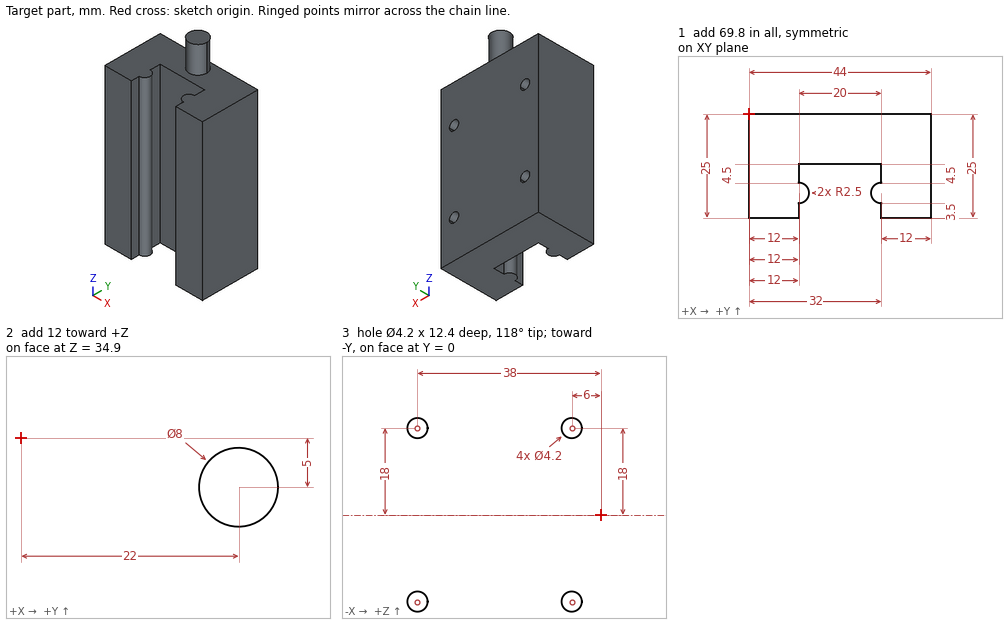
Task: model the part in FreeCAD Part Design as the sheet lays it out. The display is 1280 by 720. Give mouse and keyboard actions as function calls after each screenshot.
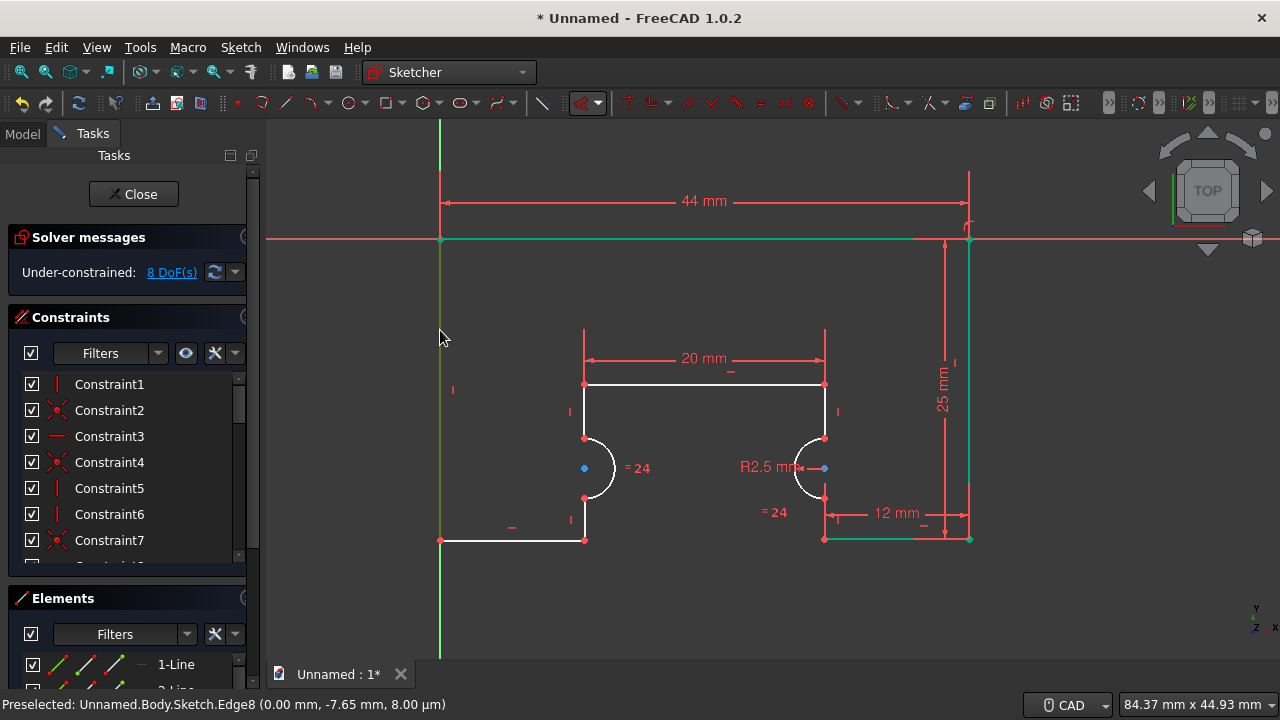
click(600, 104)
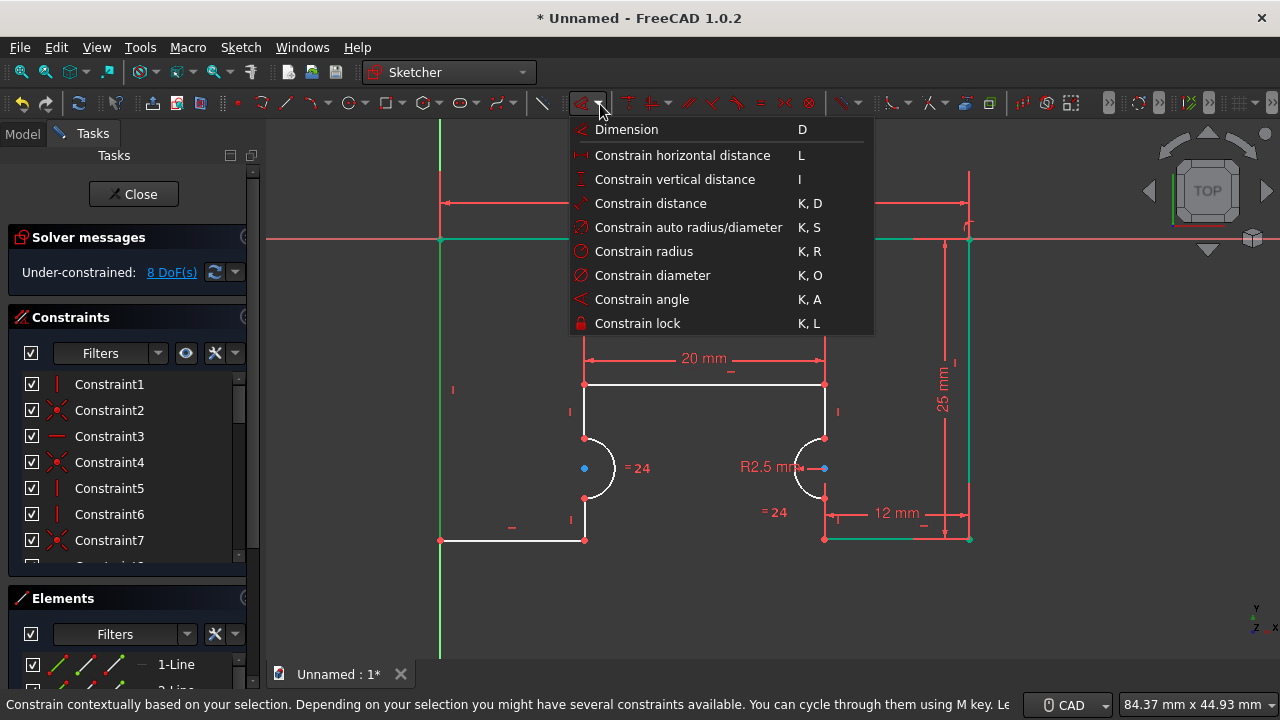
click(722, 179)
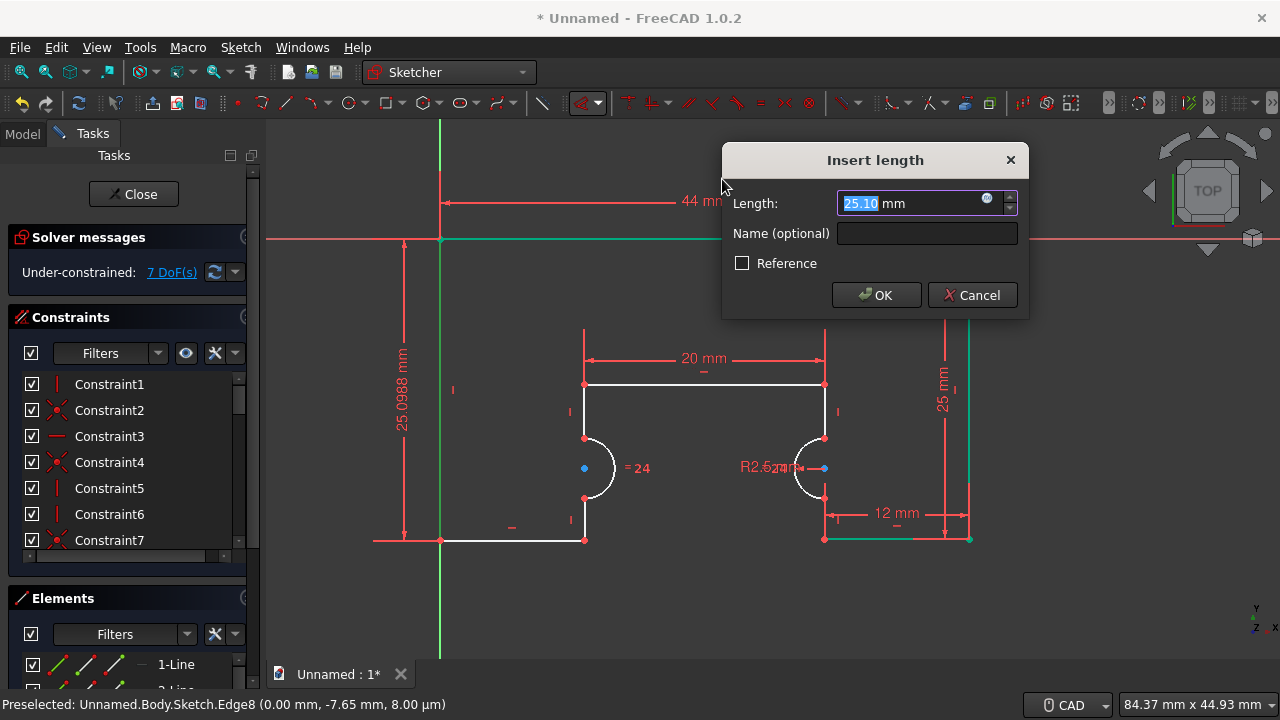
text(25)
key(Return)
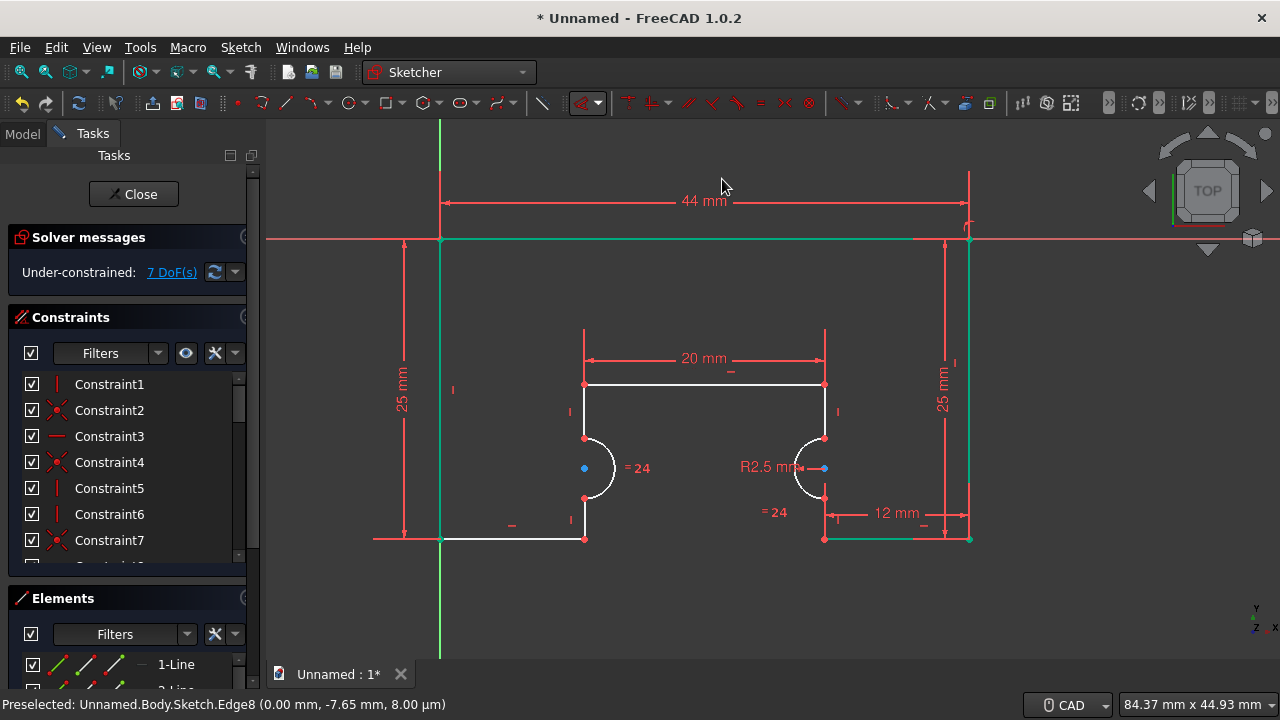
click(484, 539)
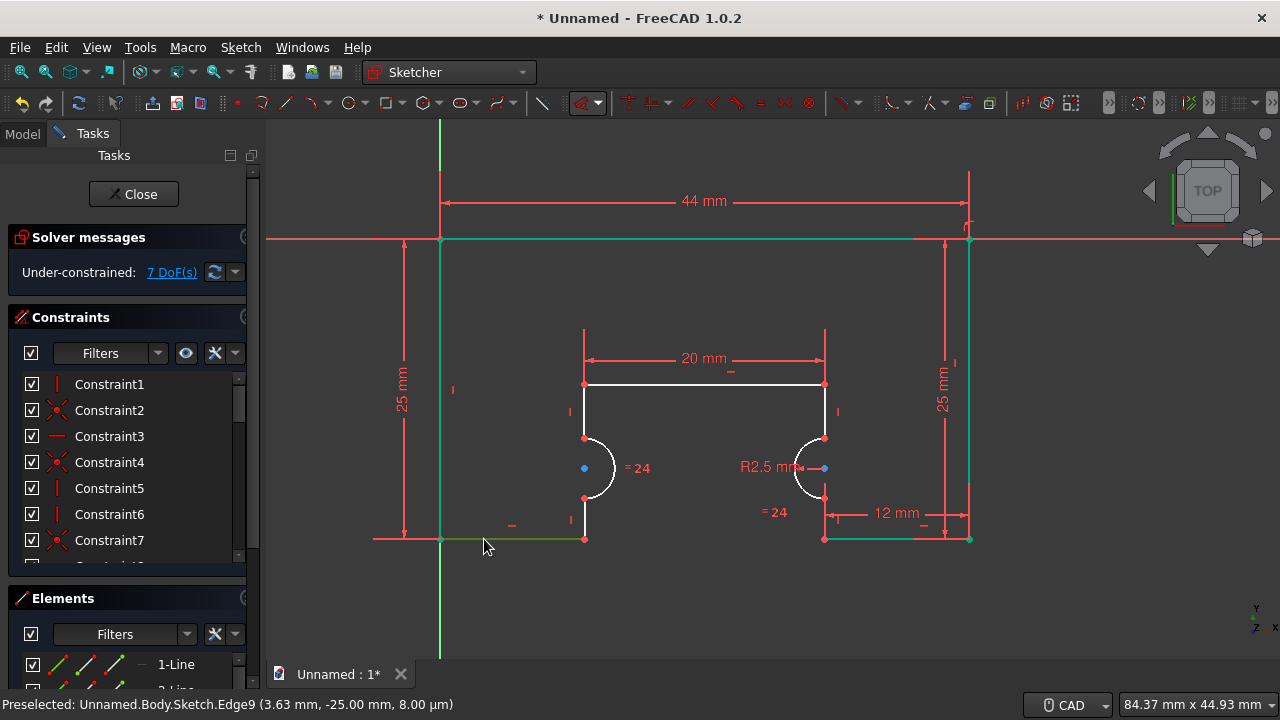
click(600, 104)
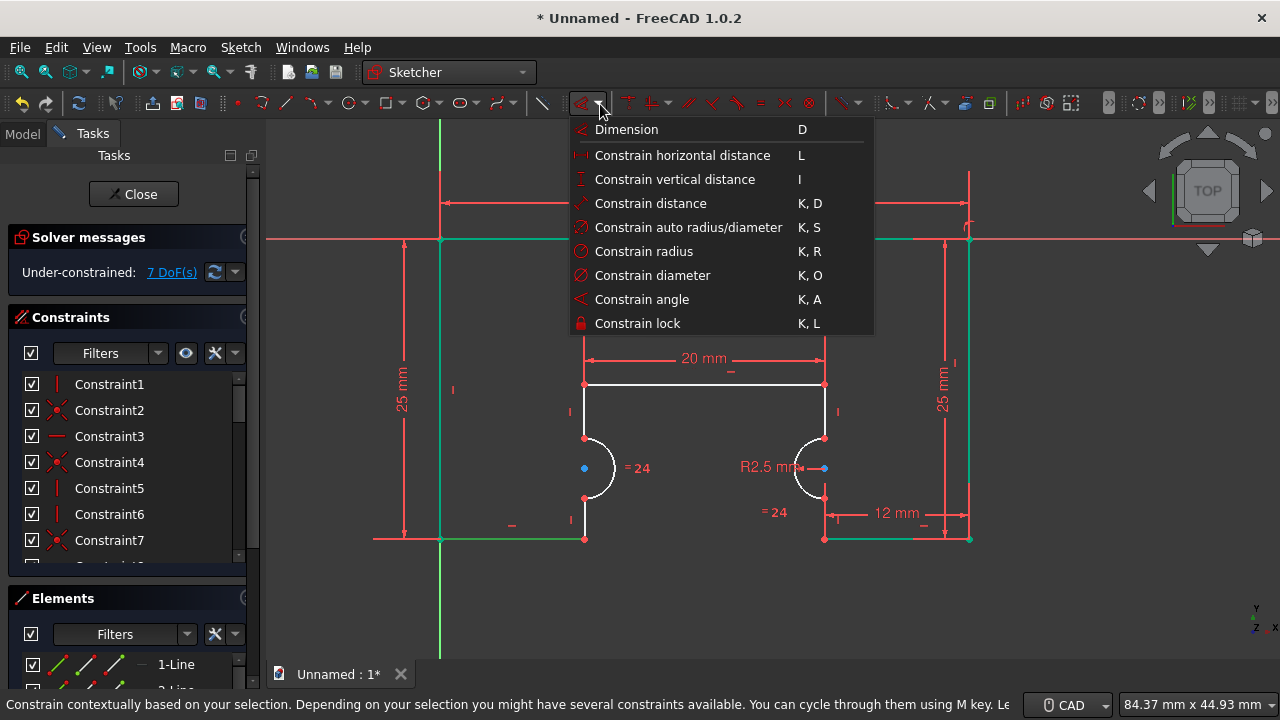
click(722, 155)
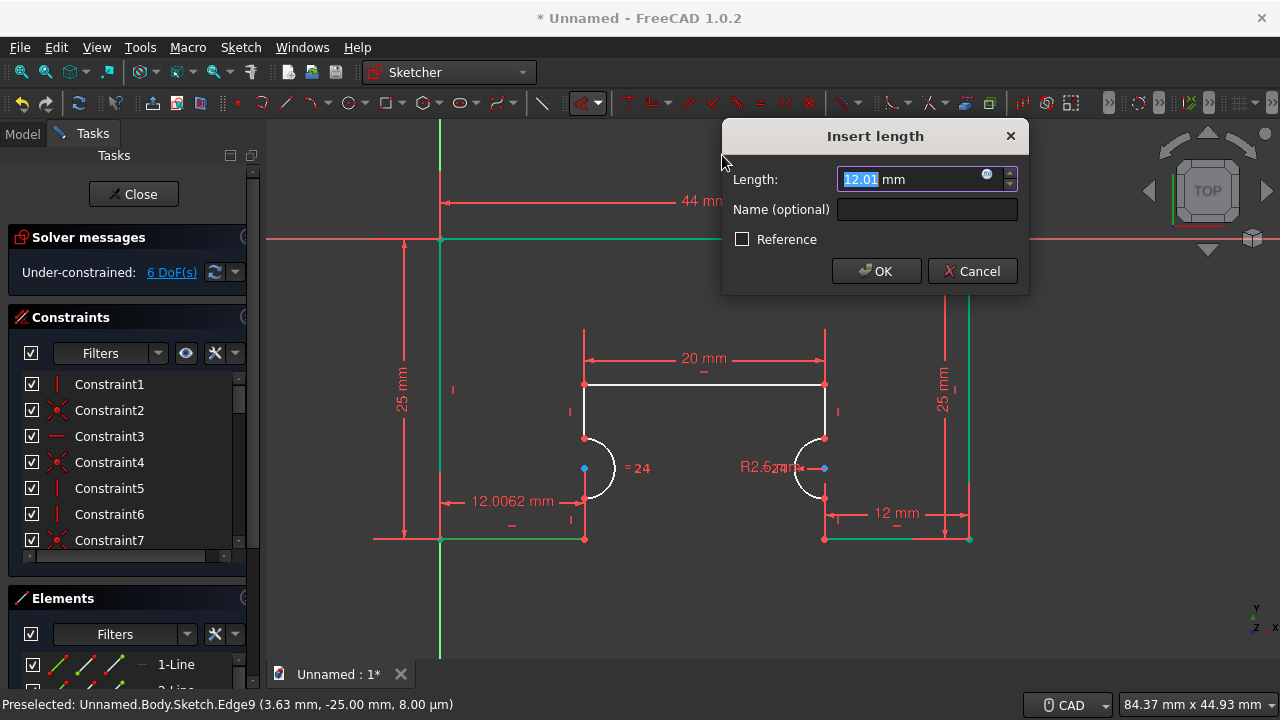
text(12)
key(Return)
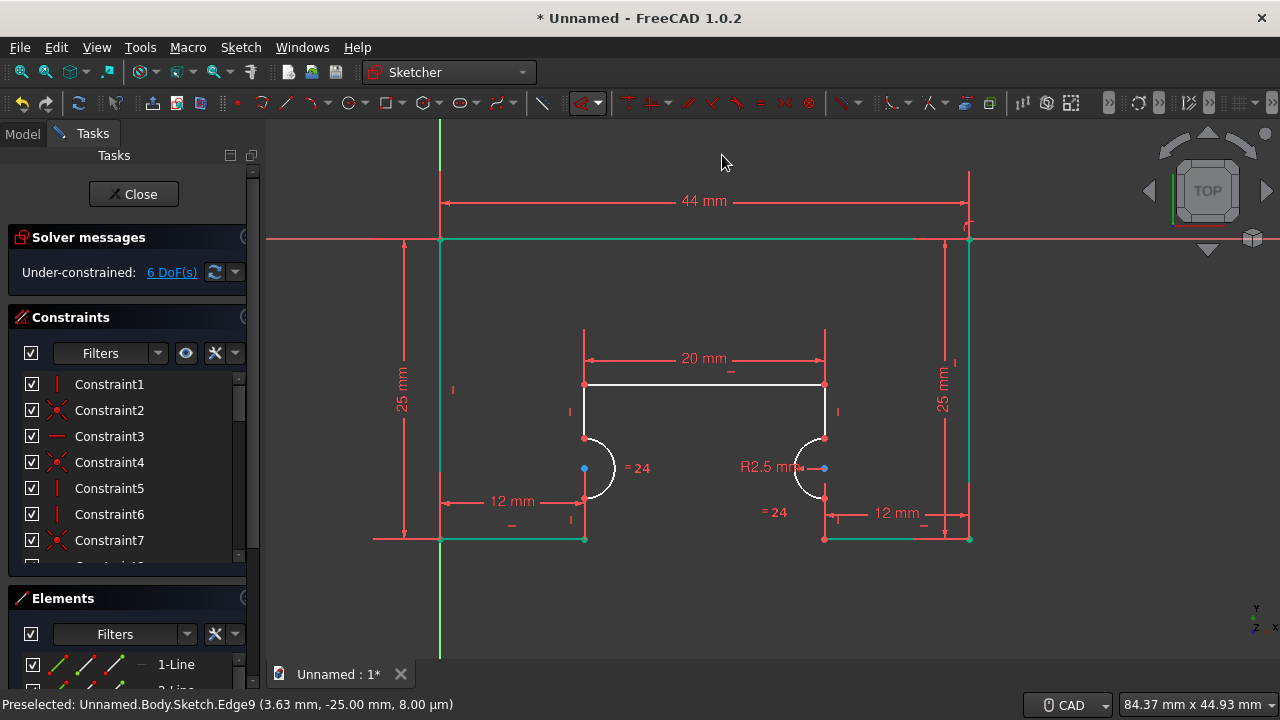
click(584, 422)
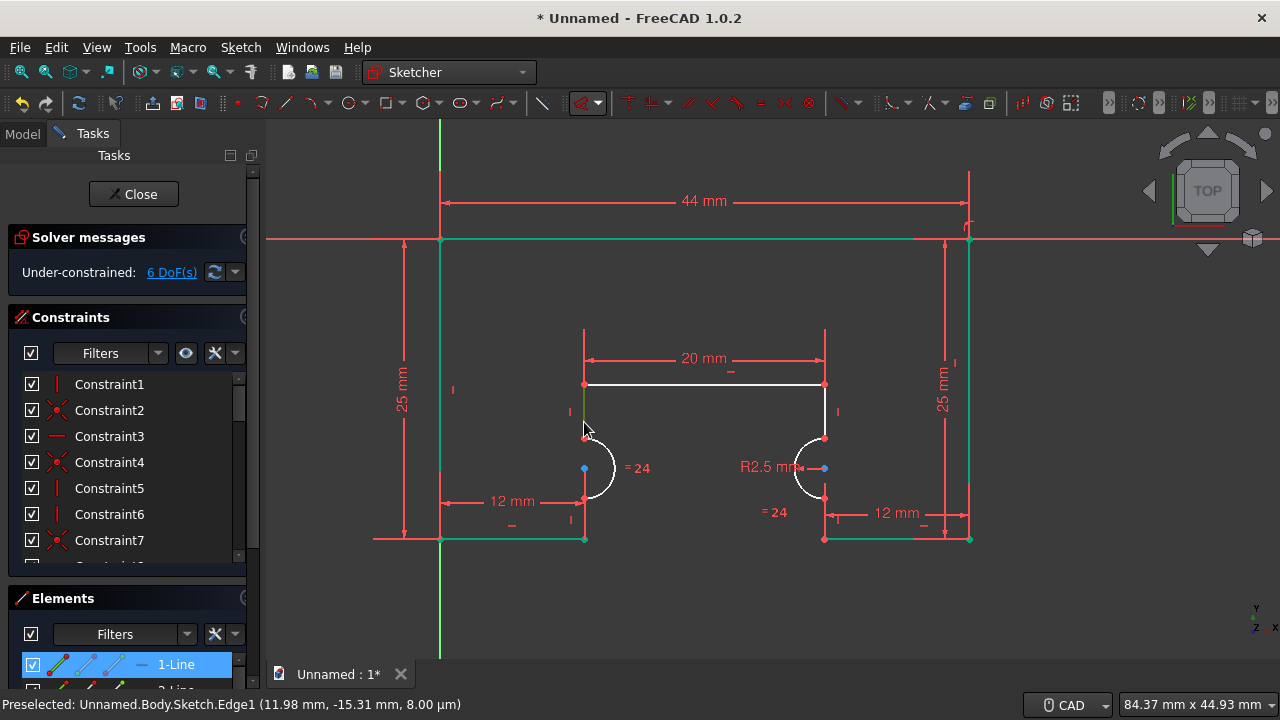
click(600, 104)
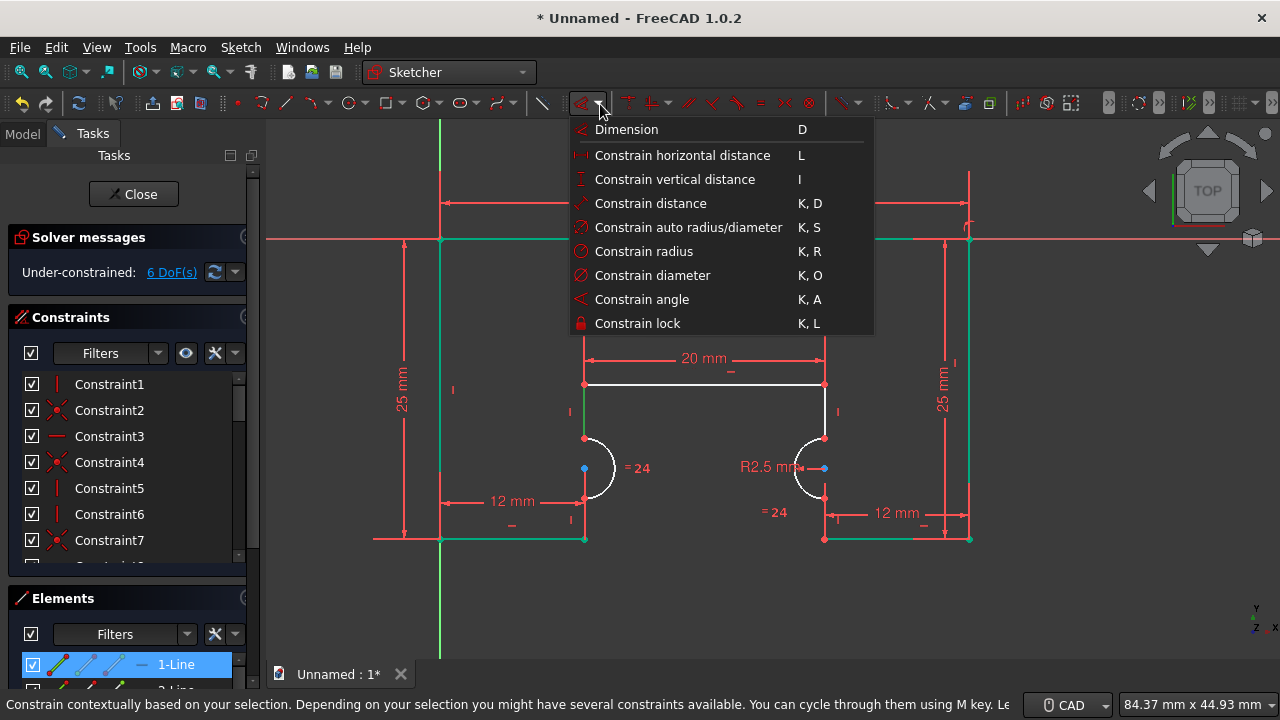
click(722, 179)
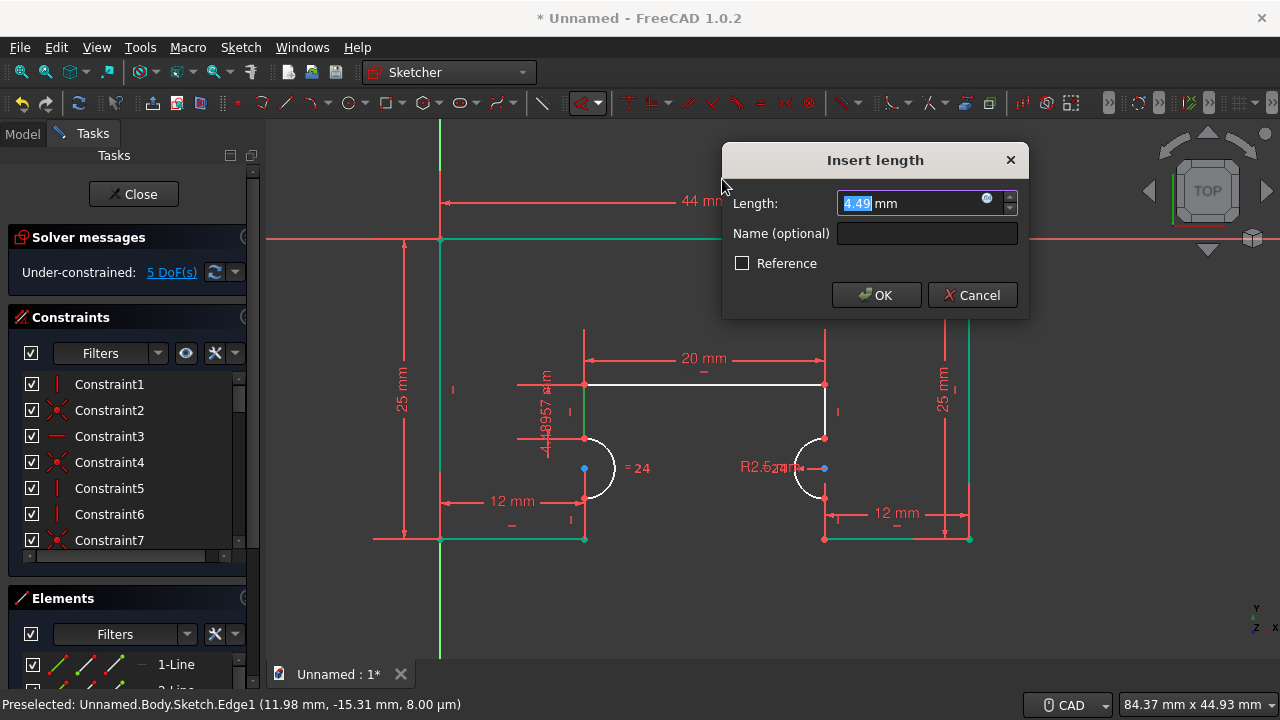
text(4.5)
key(Return)